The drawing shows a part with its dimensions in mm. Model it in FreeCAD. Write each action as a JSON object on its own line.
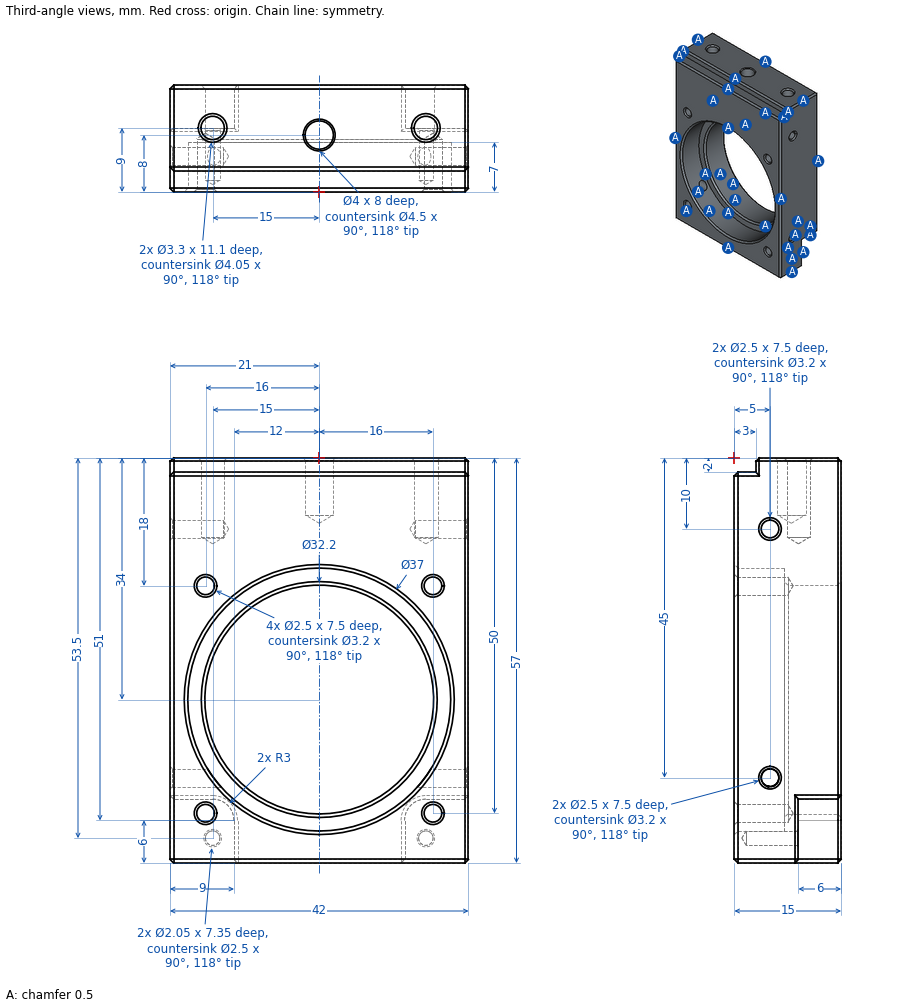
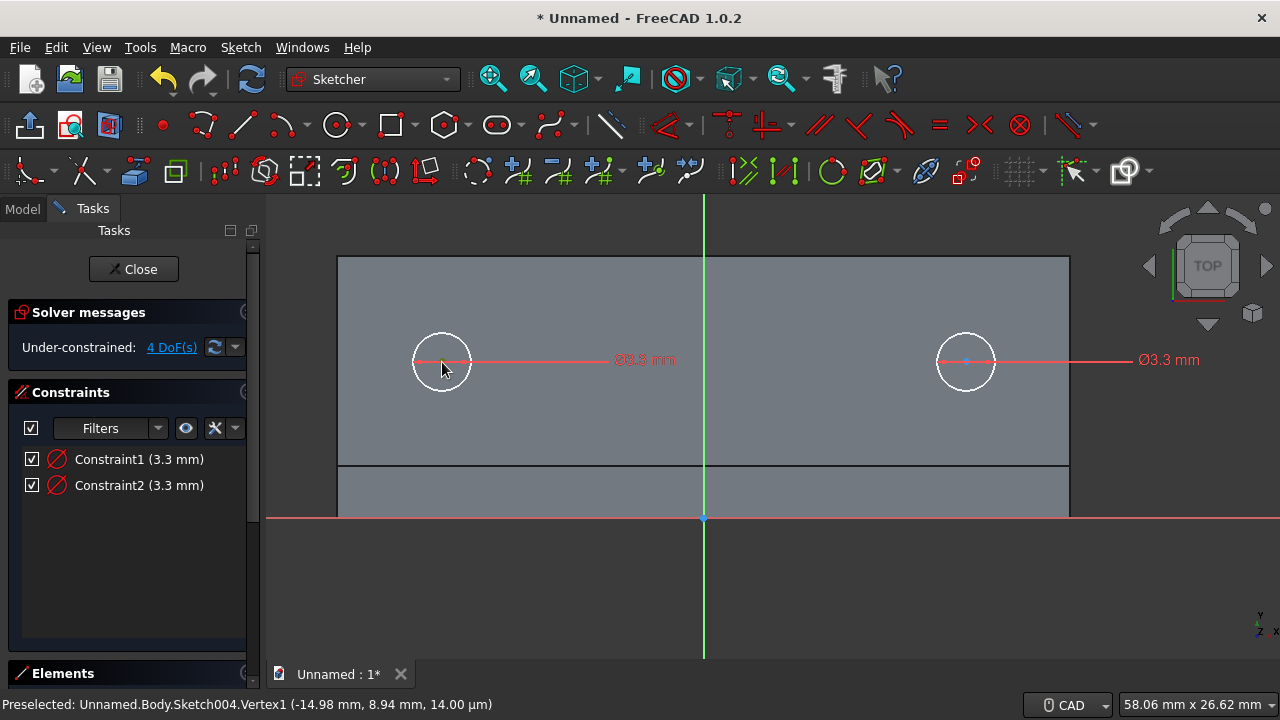
{"action": "left_click", "coordinate": [966, 362]}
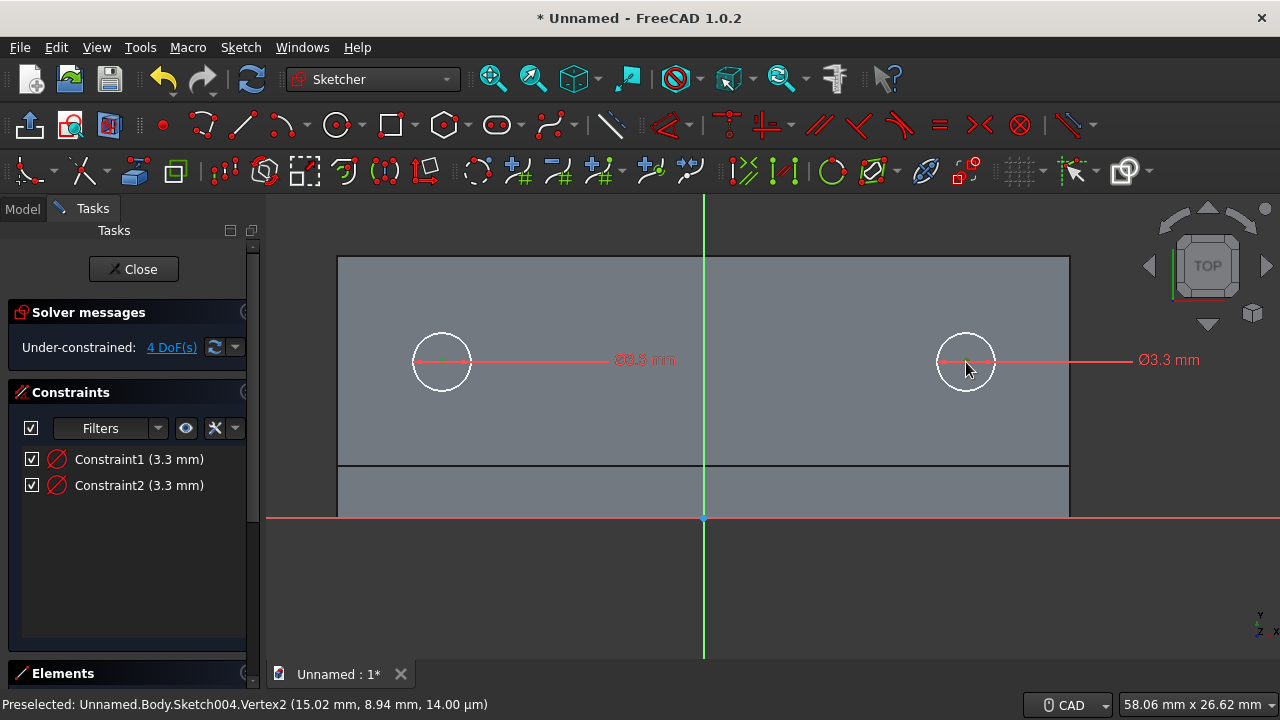
{"action": "left_click", "coordinate": [704, 602]}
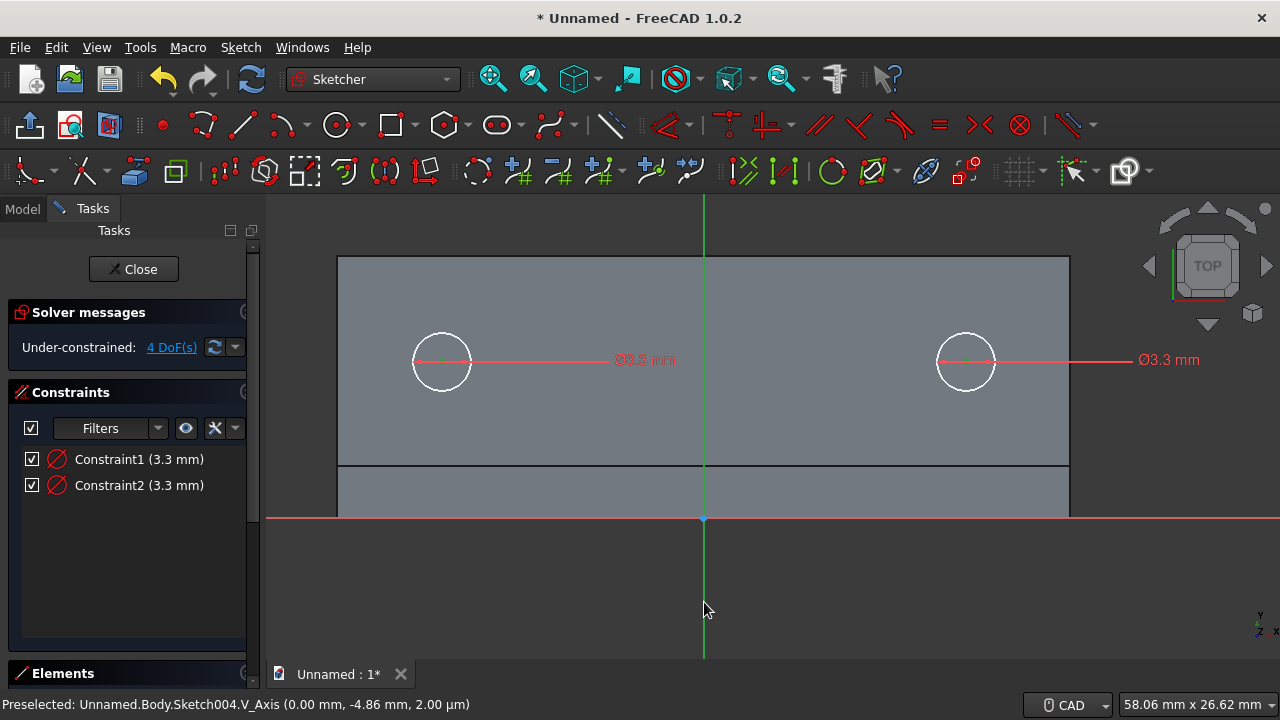
{"action": "key", "text": "s"}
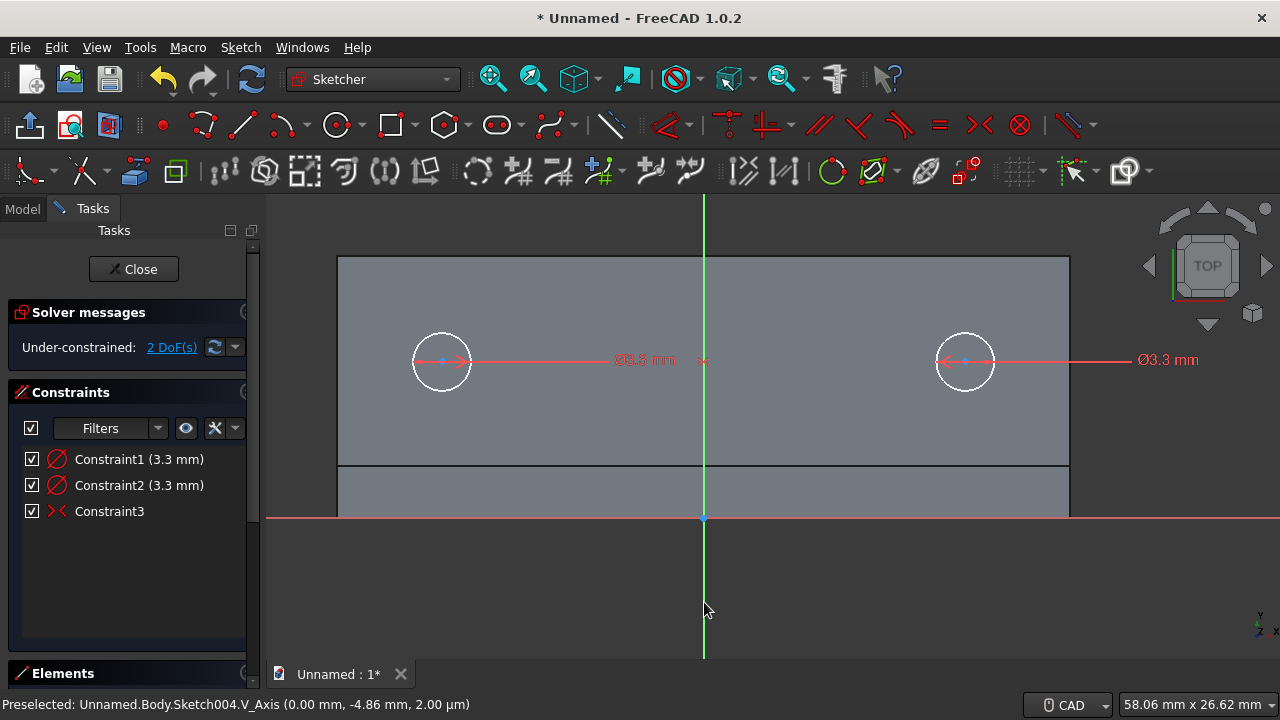
{"action": "left_click", "coordinate": [666, 126]}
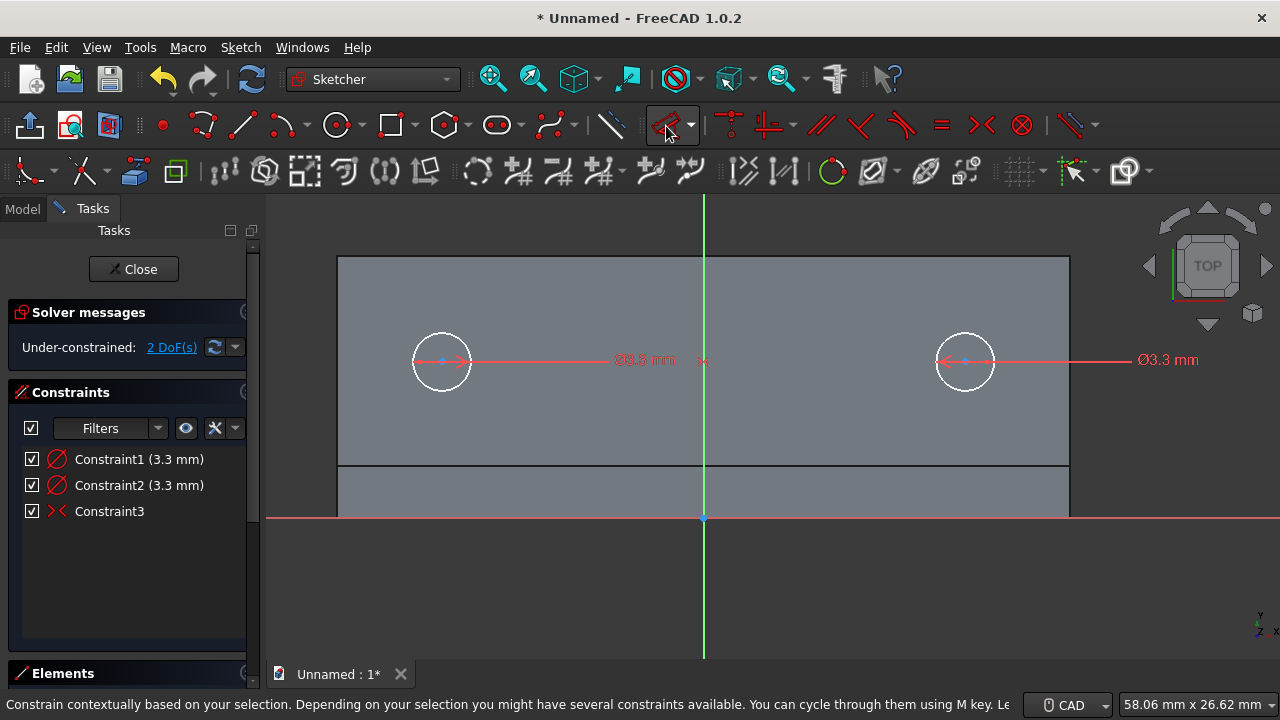
{"action": "left_click", "coordinate": [442, 362]}
{"action": "left_click", "coordinate": [408, 440]}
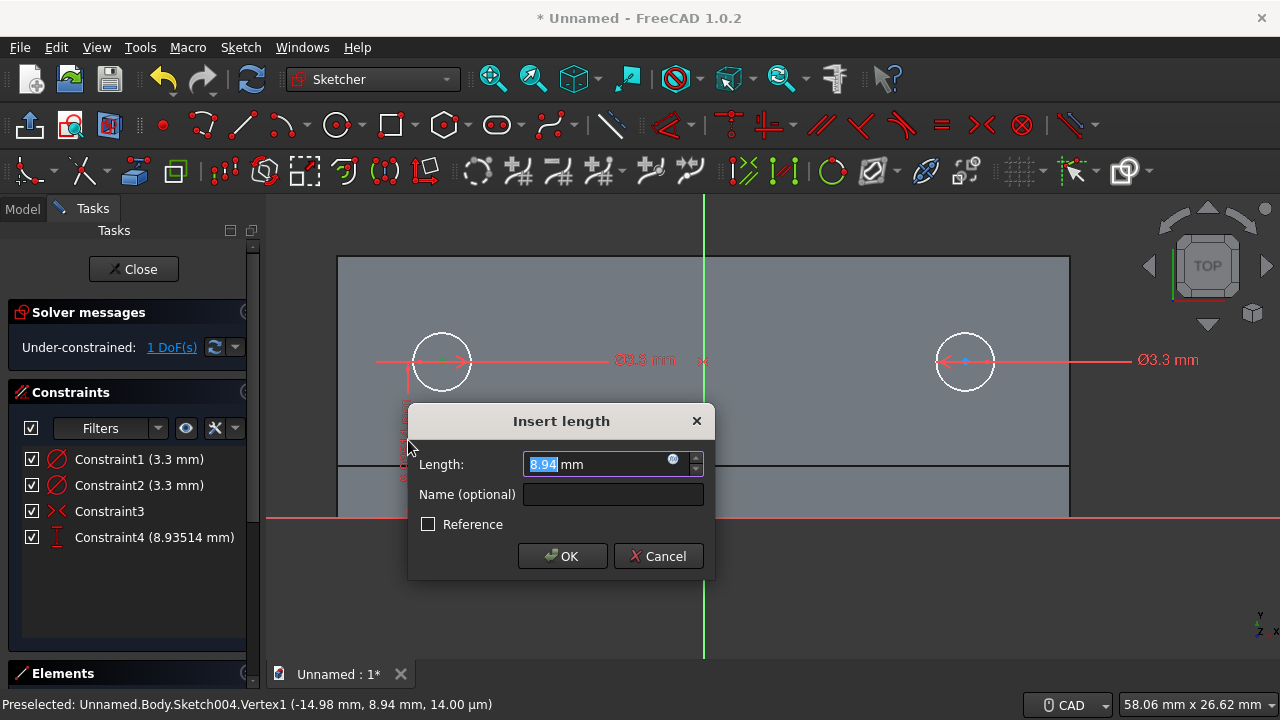
{"action": "type", "text": "9"}
{"action": "key", "text": "Return"}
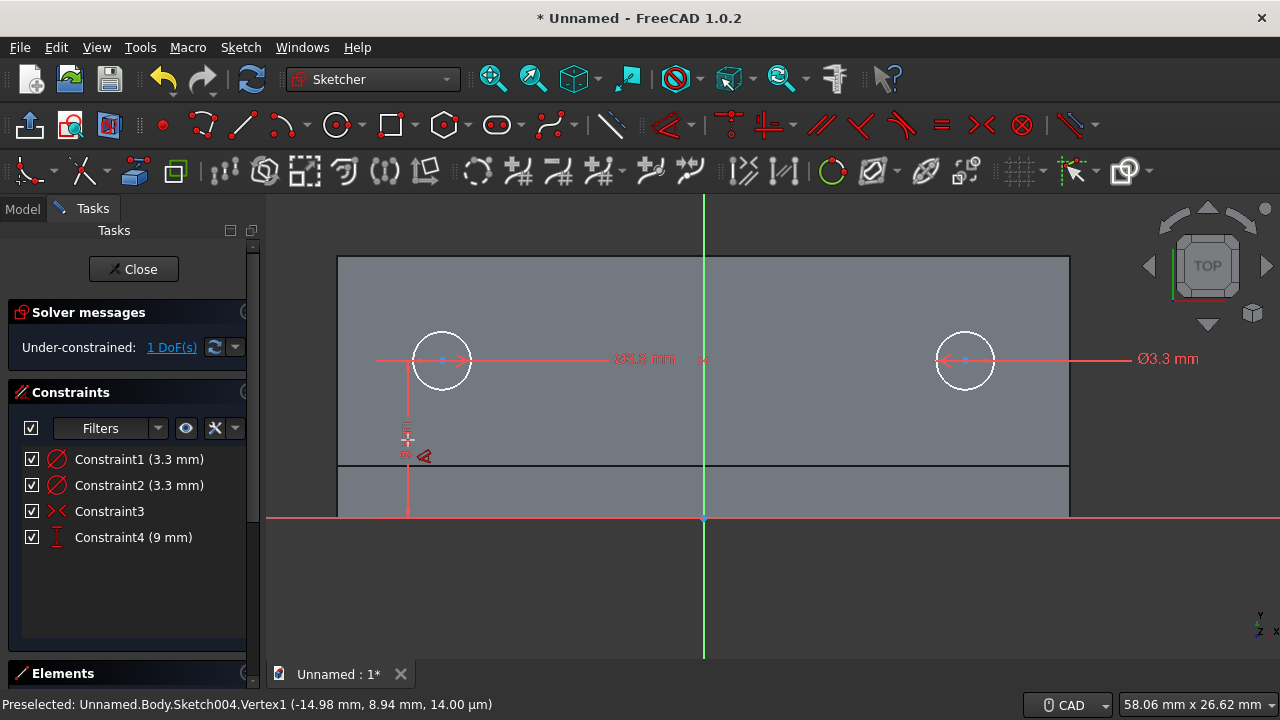
{"action": "left_click", "coordinate": [442, 361]}
{"action": "left_click", "coordinate": [573, 552]}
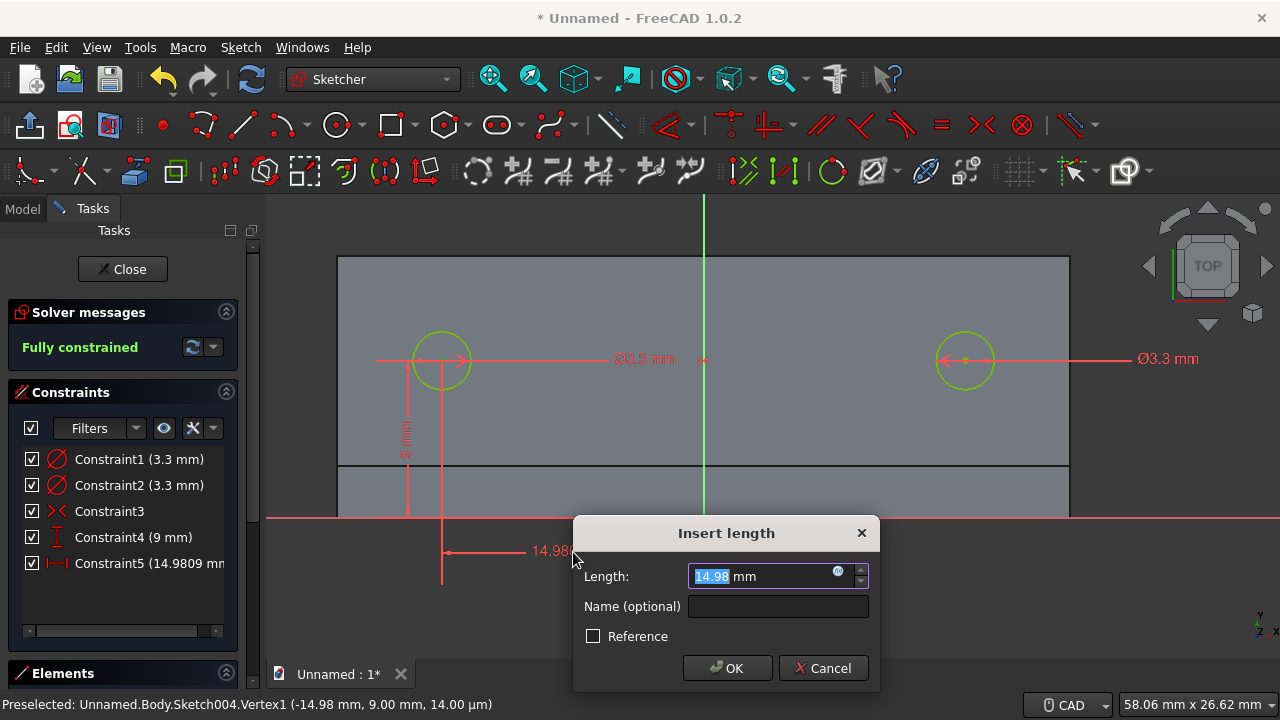
{"action": "type", "text": "15"}
{"action": "key", "text": "Return"}
{"action": "key", "text": "Escape"}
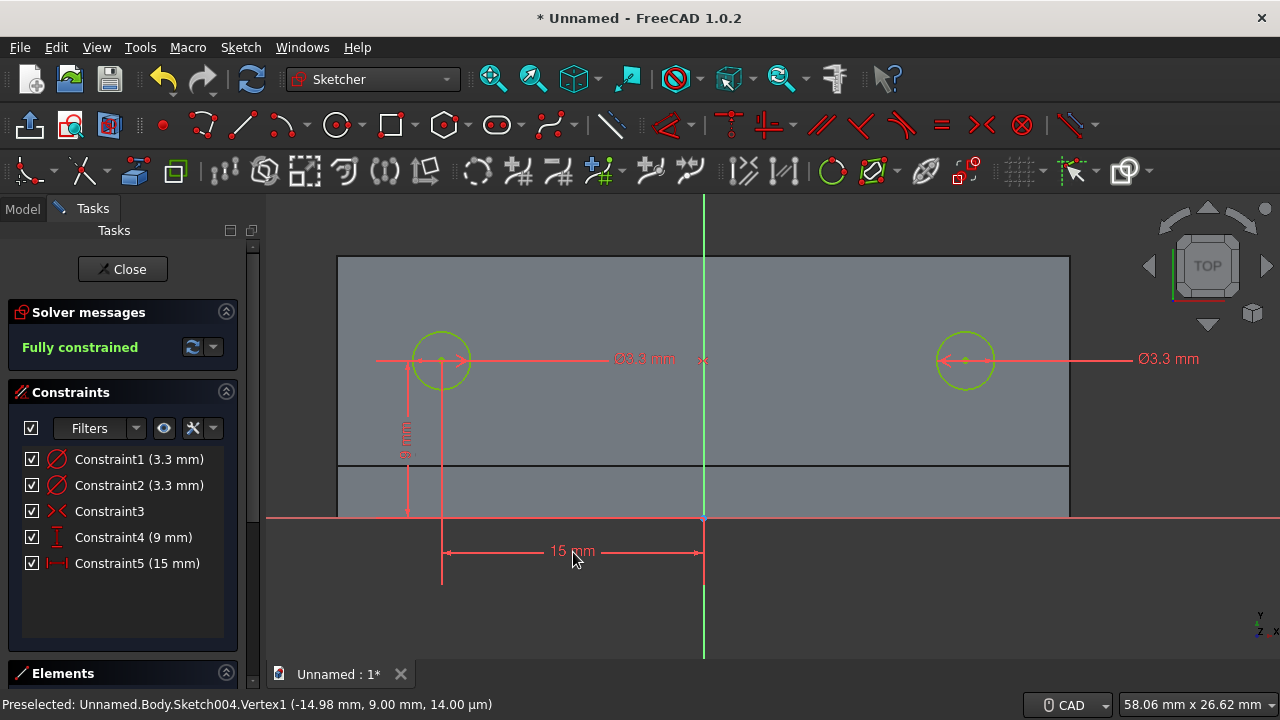
{"action": "left_click", "coordinate": [123, 269]}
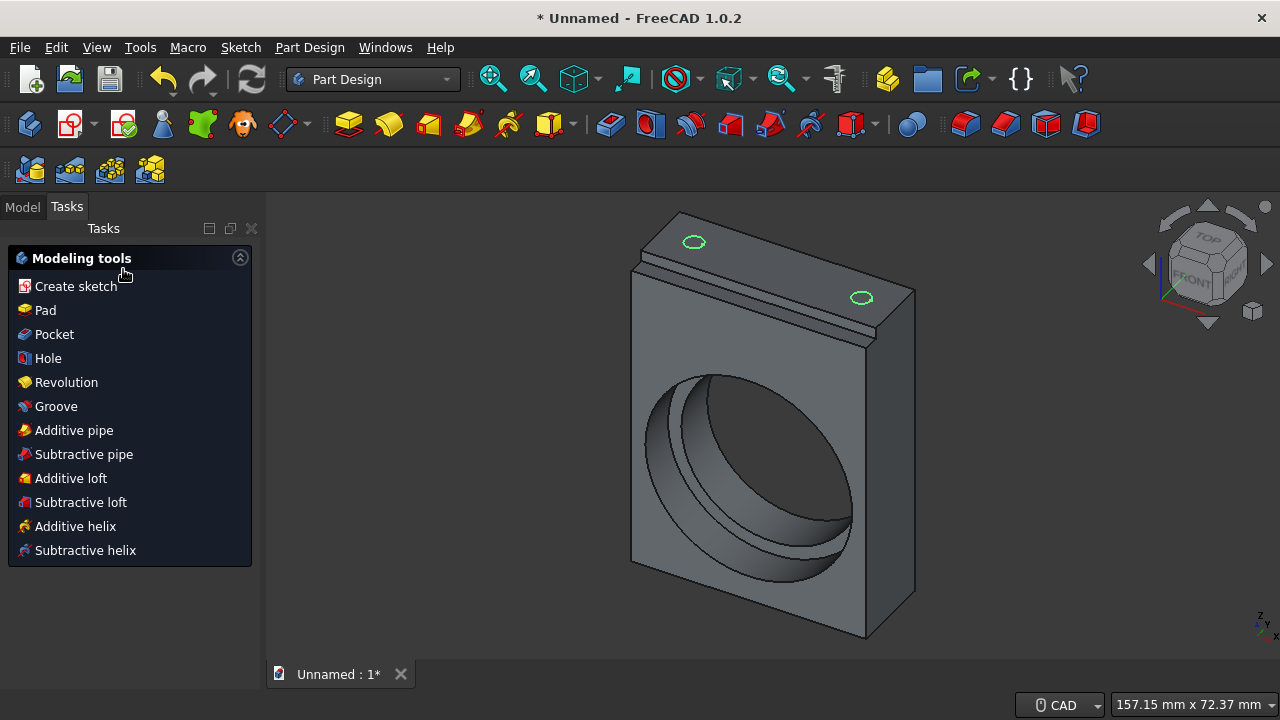
{"action": "left_click", "coordinate": [652, 124]}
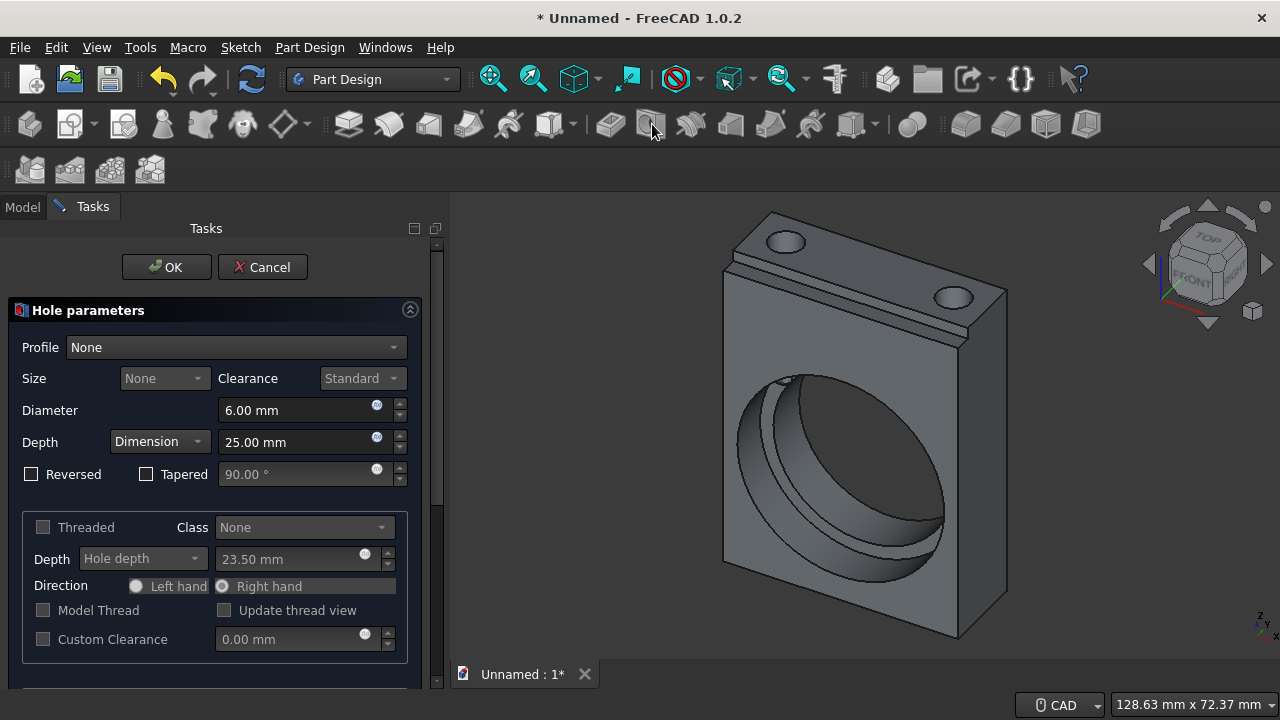
{"action": "triple_click", "coordinate": [305, 410]}